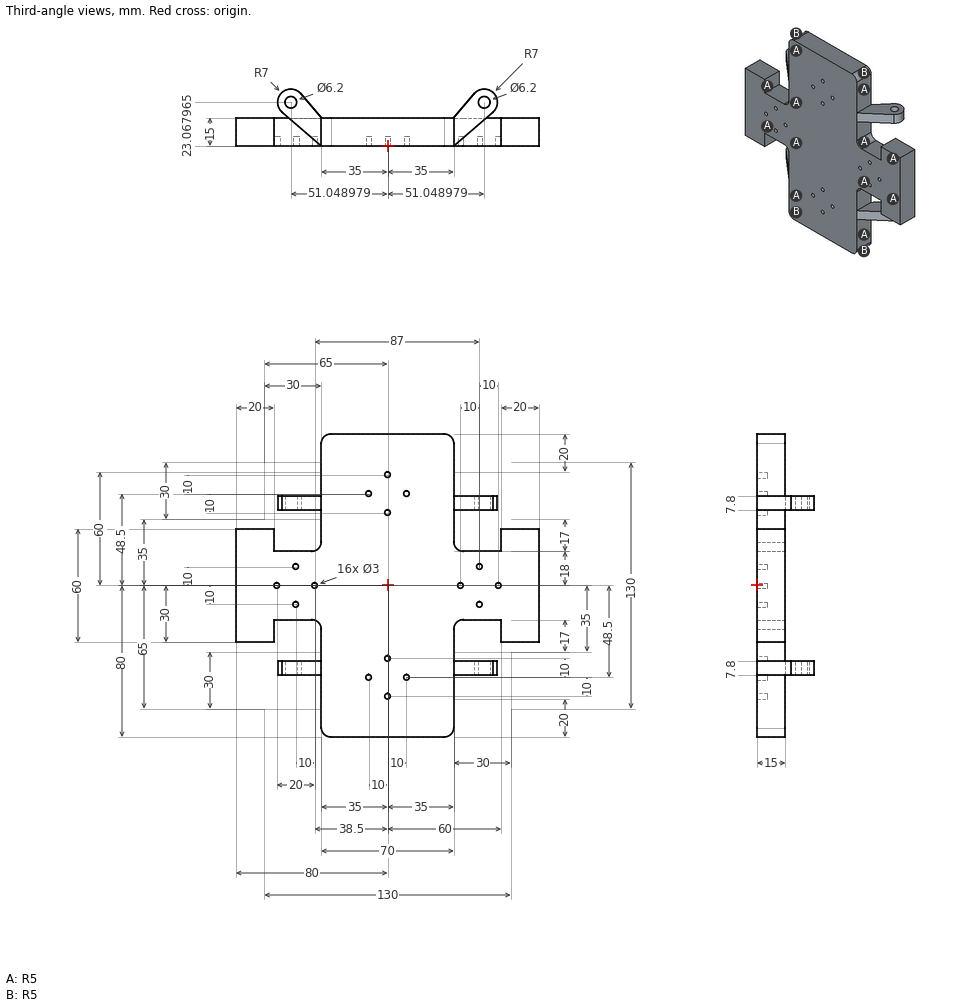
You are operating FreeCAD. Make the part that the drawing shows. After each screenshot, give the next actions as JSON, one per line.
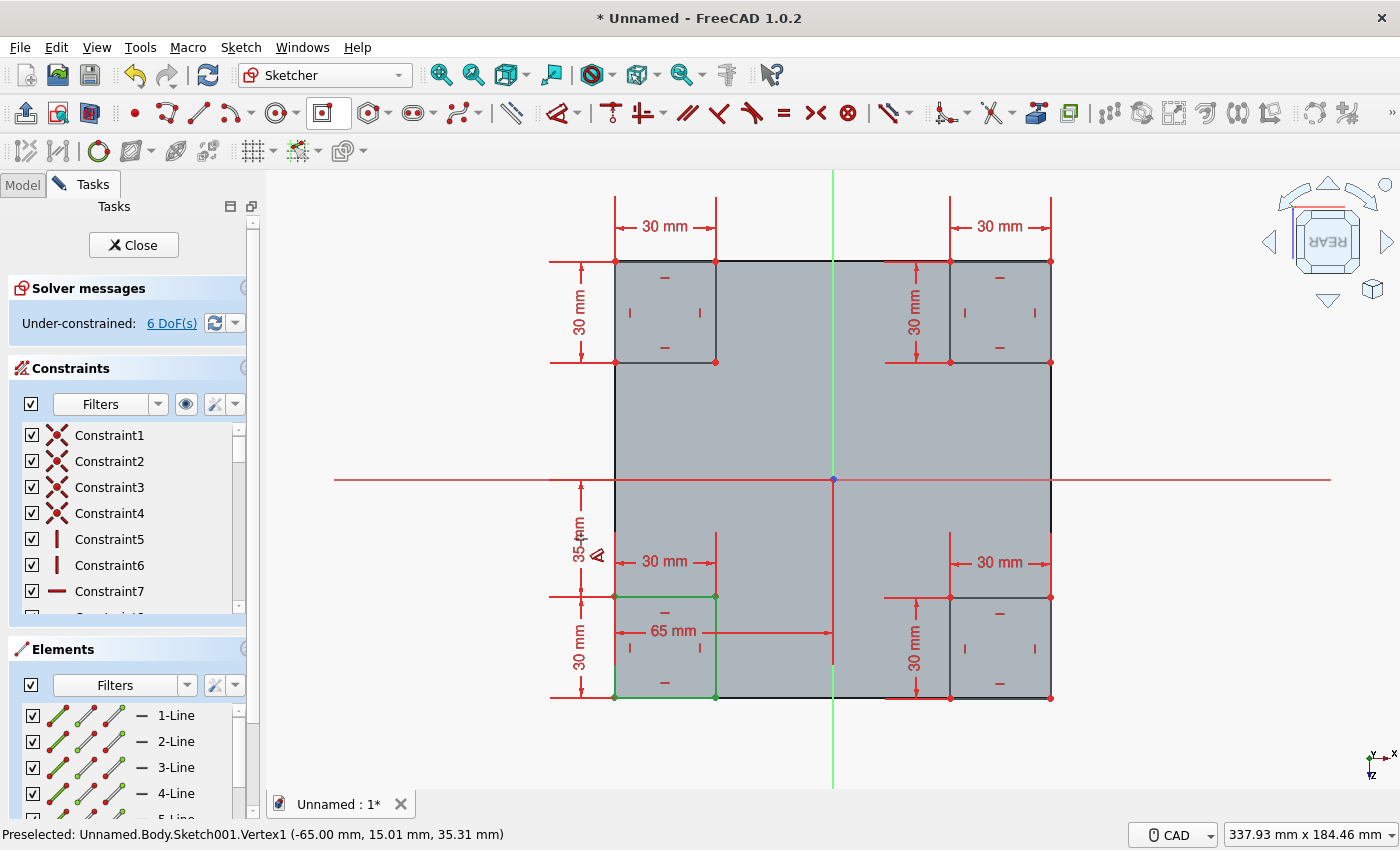
{"action": "left_click", "coordinate": [615, 262]}
{"action": "left_click", "coordinate": [724, 228]}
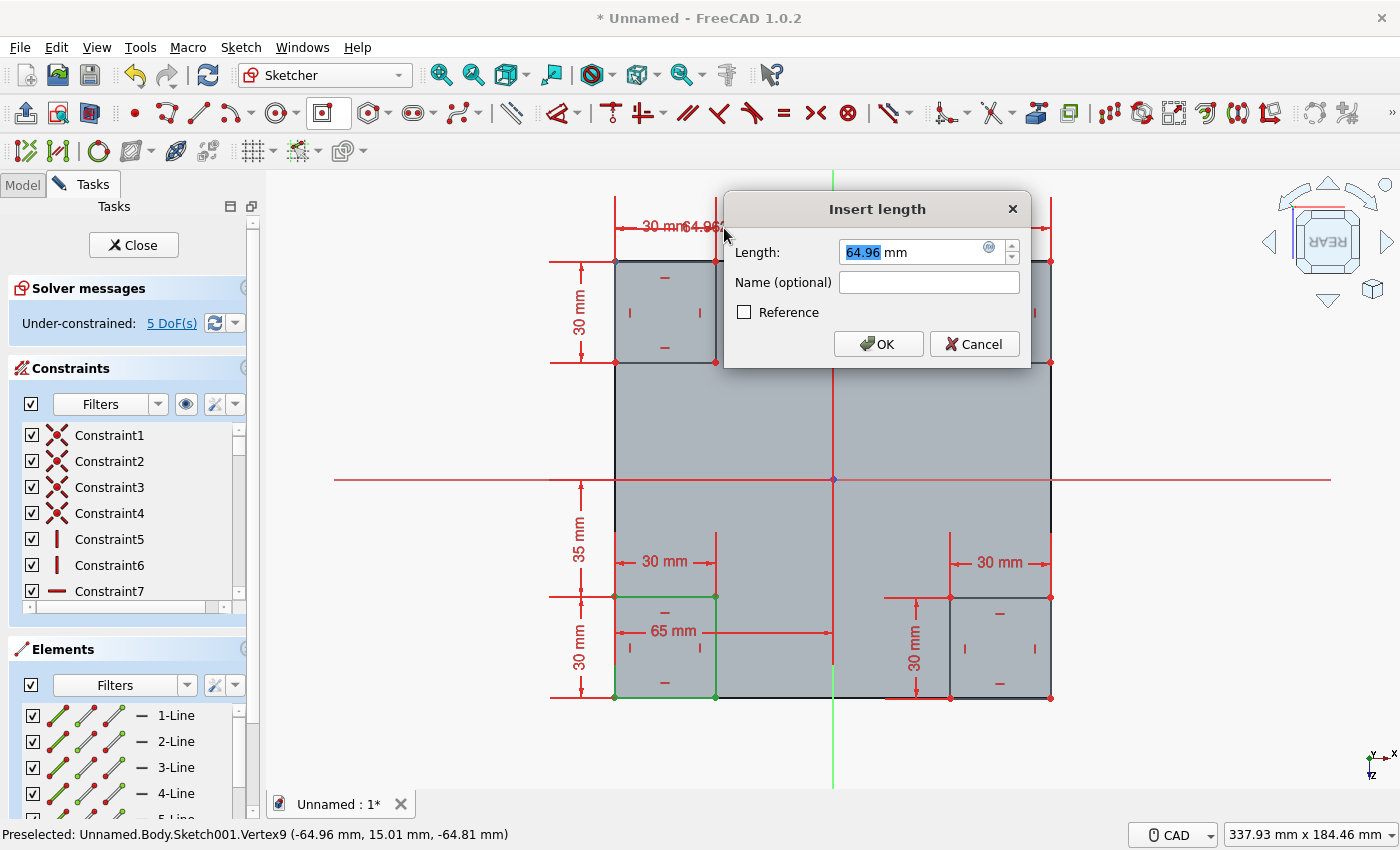
{"action": "type", "text": "65"}
{"action": "key", "text": "Return"}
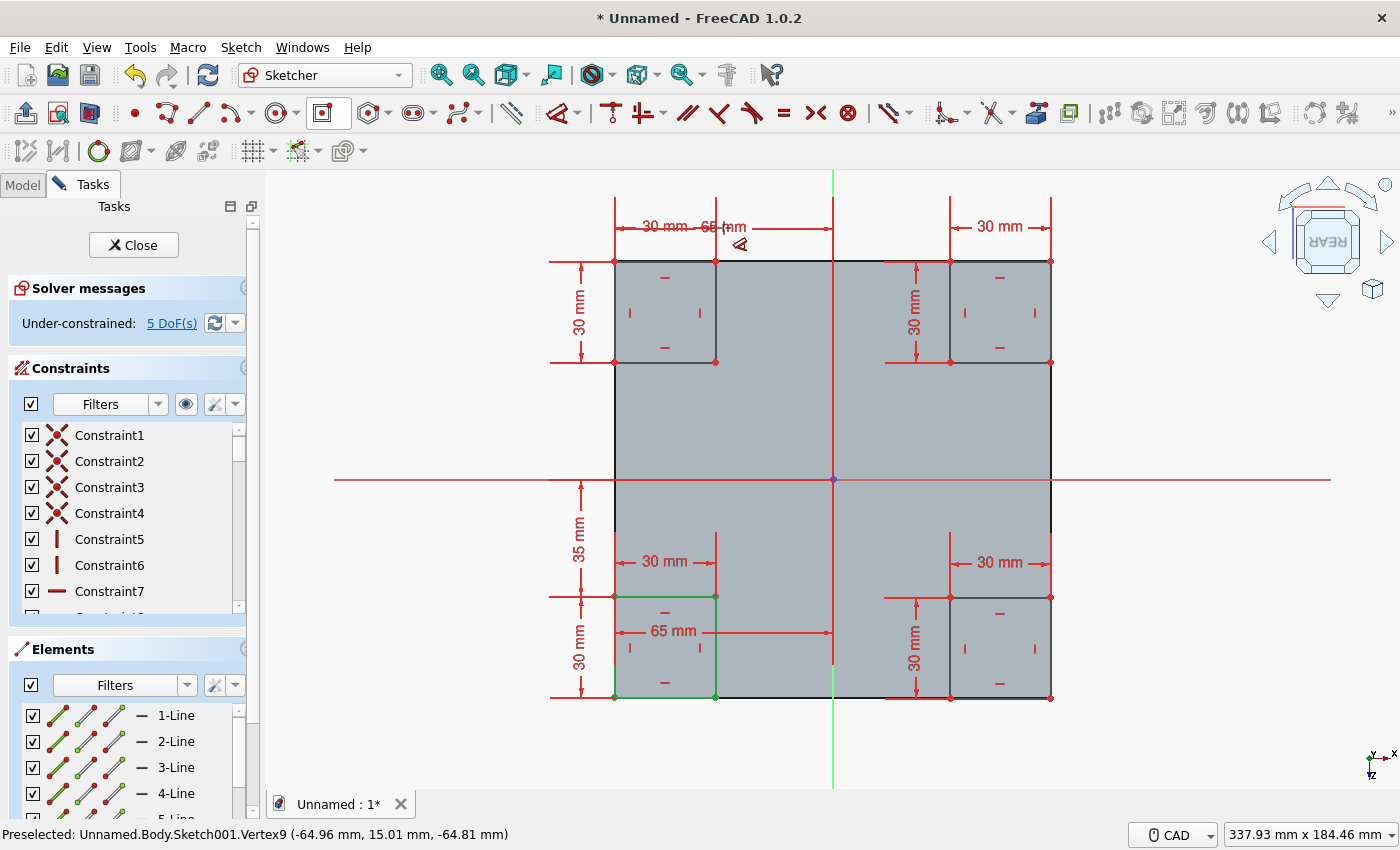
{"action": "left_click", "coordinate": [615, 262]}
{"action": "left_click", "coordinate": [581, 371]}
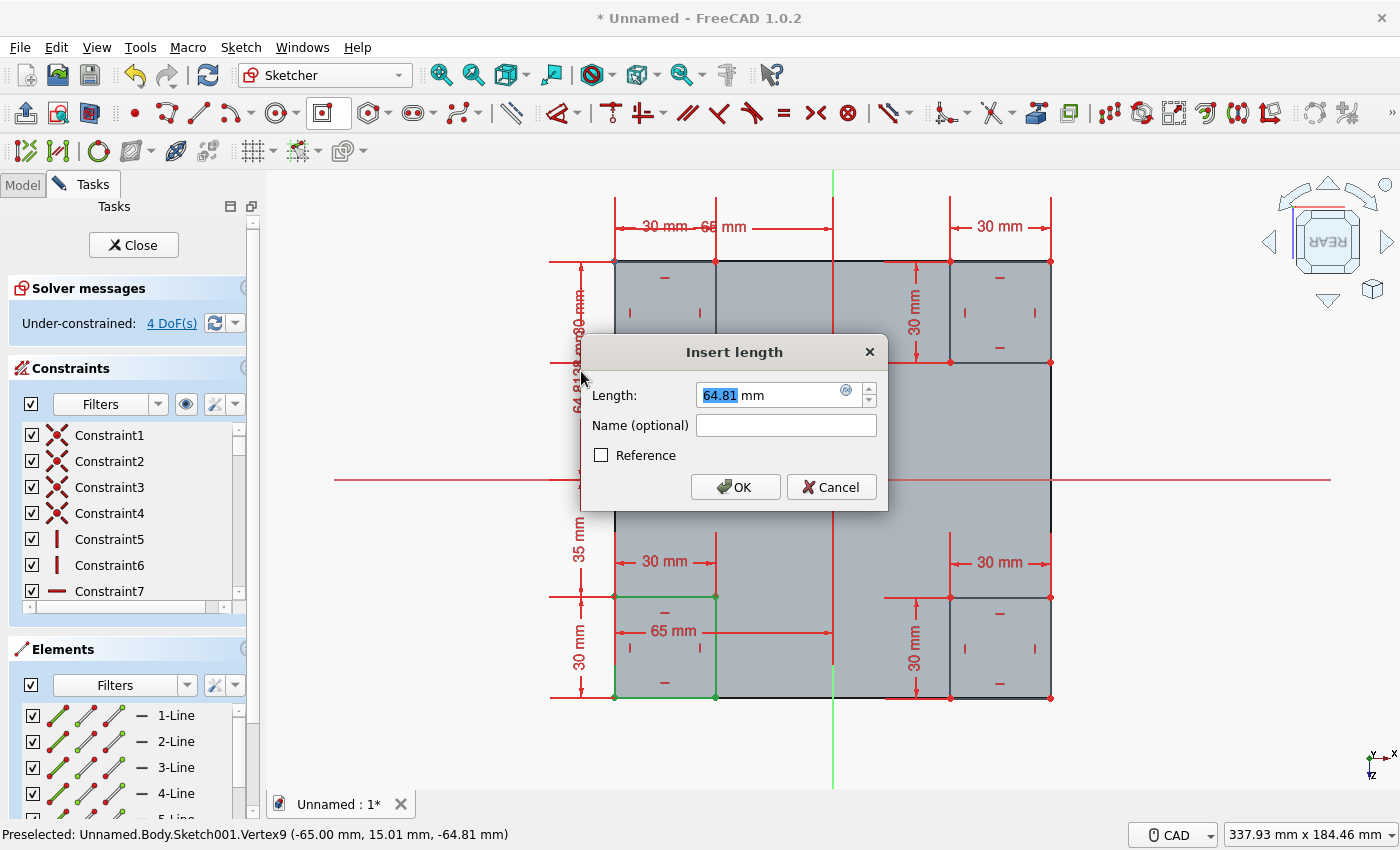
{"action": "type", "text": "65"}
{"action": "key", "text": "Return"}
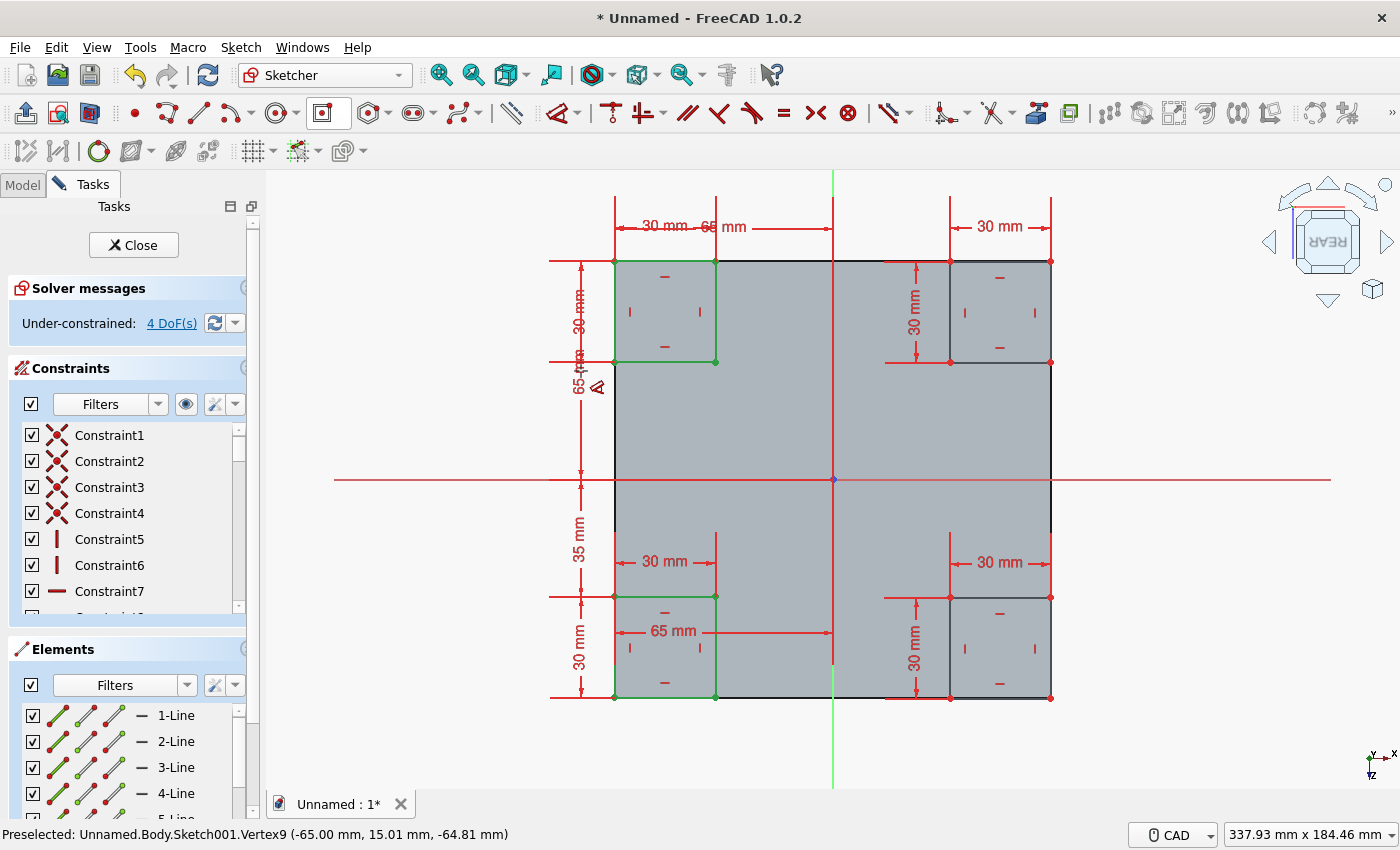
{"action": "left_click", "coordinate": [950, 262]}
{"action": "left_click", "coordinate": [892, 228]}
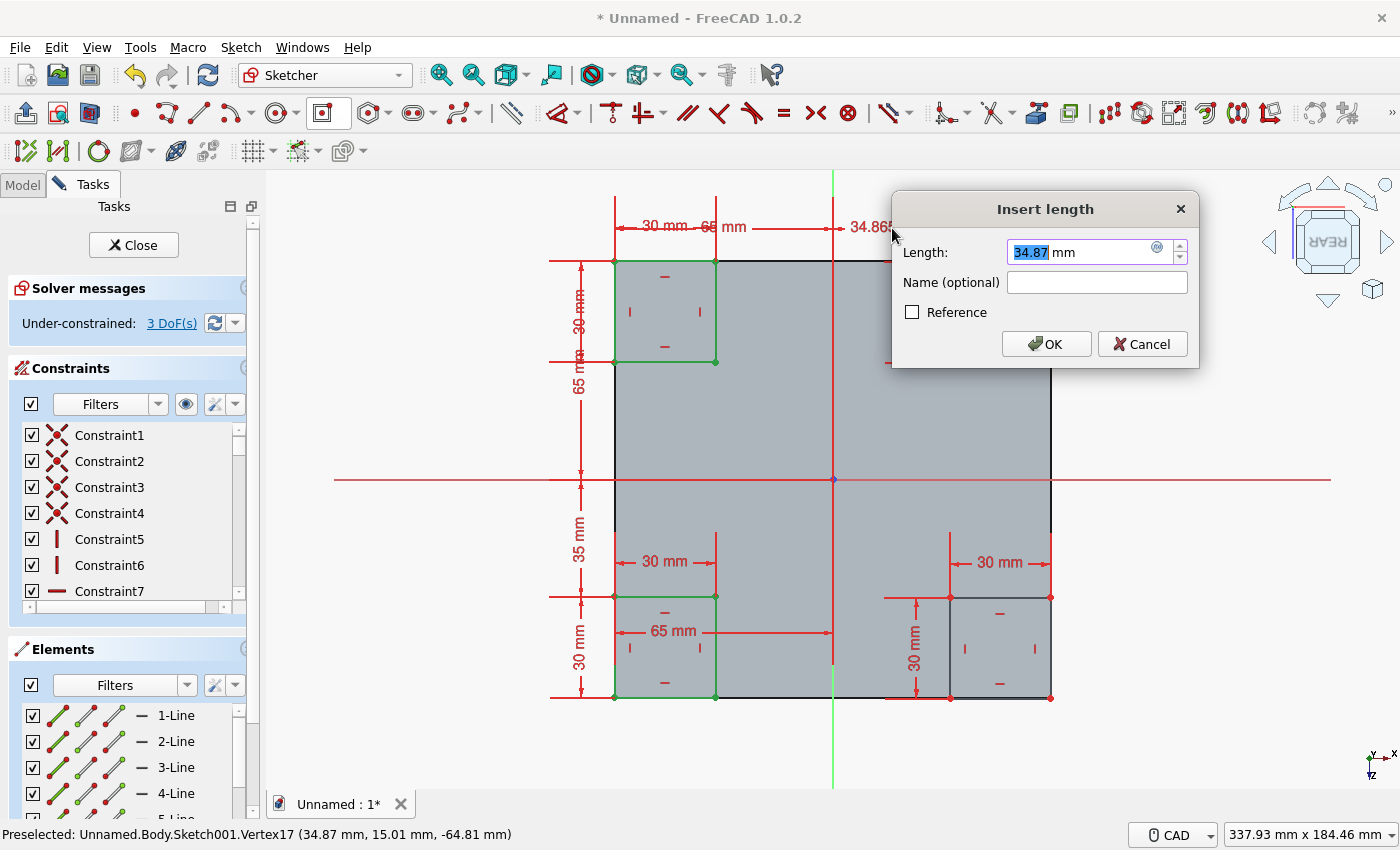
{"action": "type", "text": "35"}
{"action": "key", "text": "Return"}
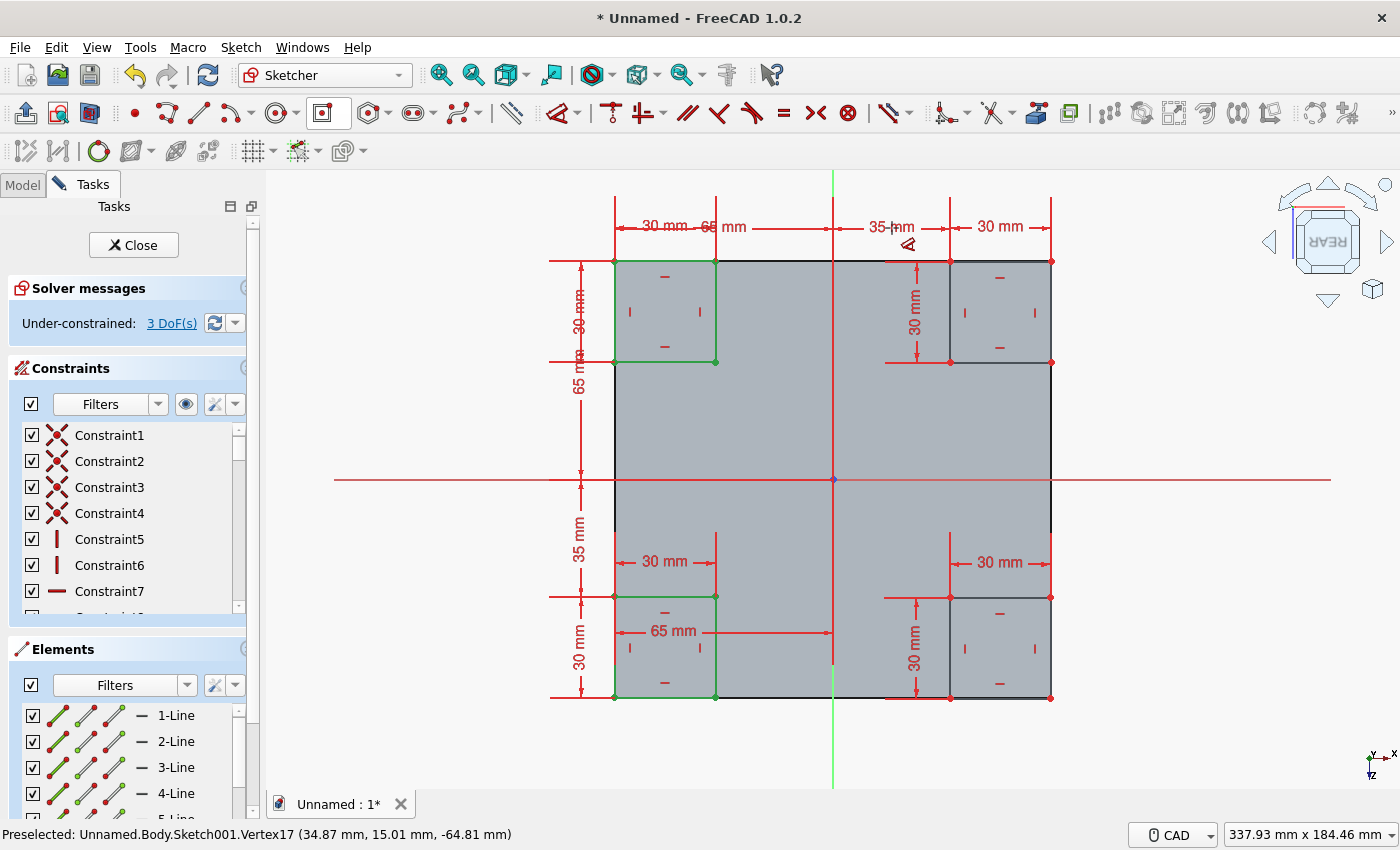
{"action": "left_click", "coordinate": [950, 262]}
{"action": "left_click", "coordinate": [984, 321]}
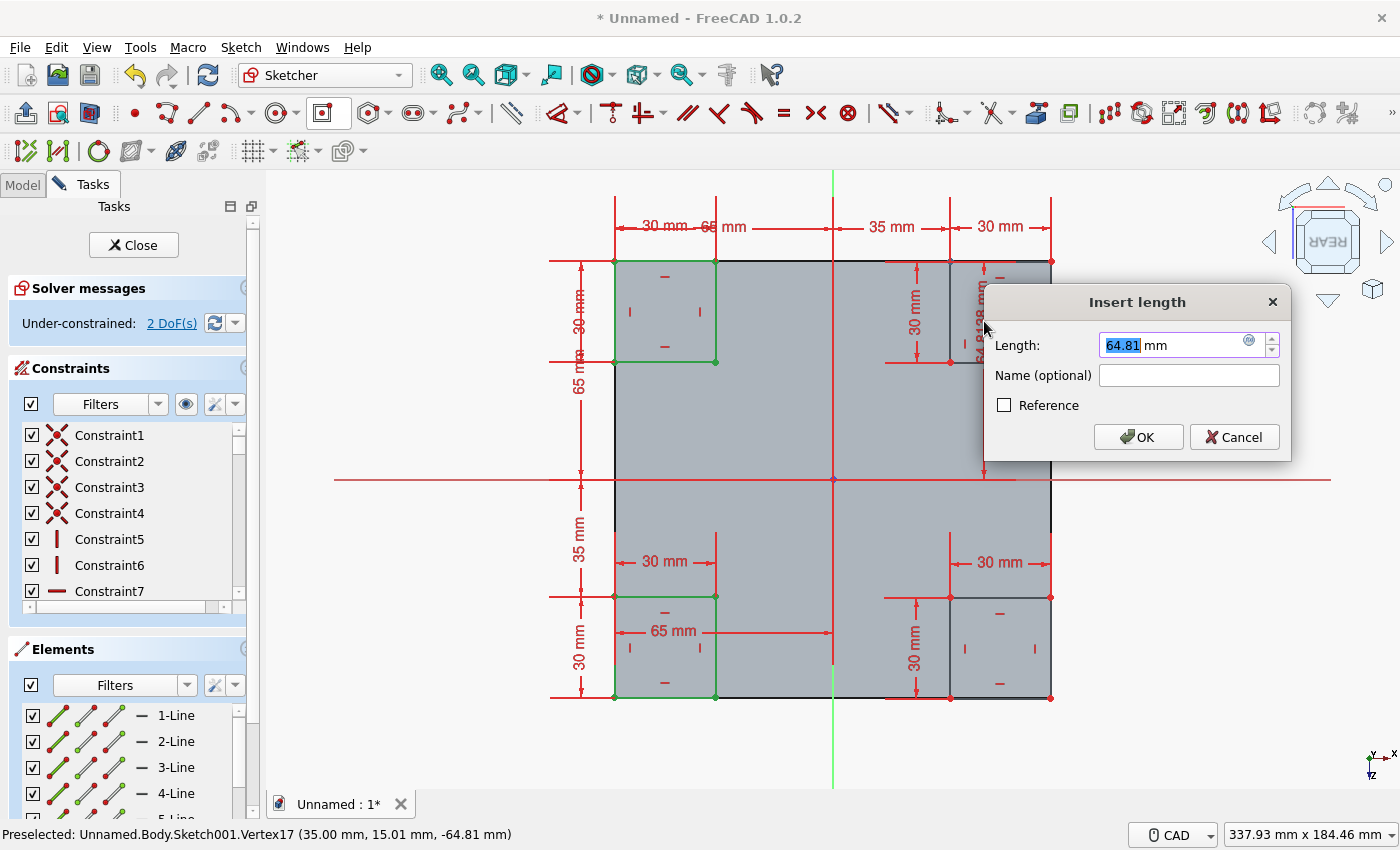
{"action": "type", "text": "65"}
{"action": "key", "text": "Return"}